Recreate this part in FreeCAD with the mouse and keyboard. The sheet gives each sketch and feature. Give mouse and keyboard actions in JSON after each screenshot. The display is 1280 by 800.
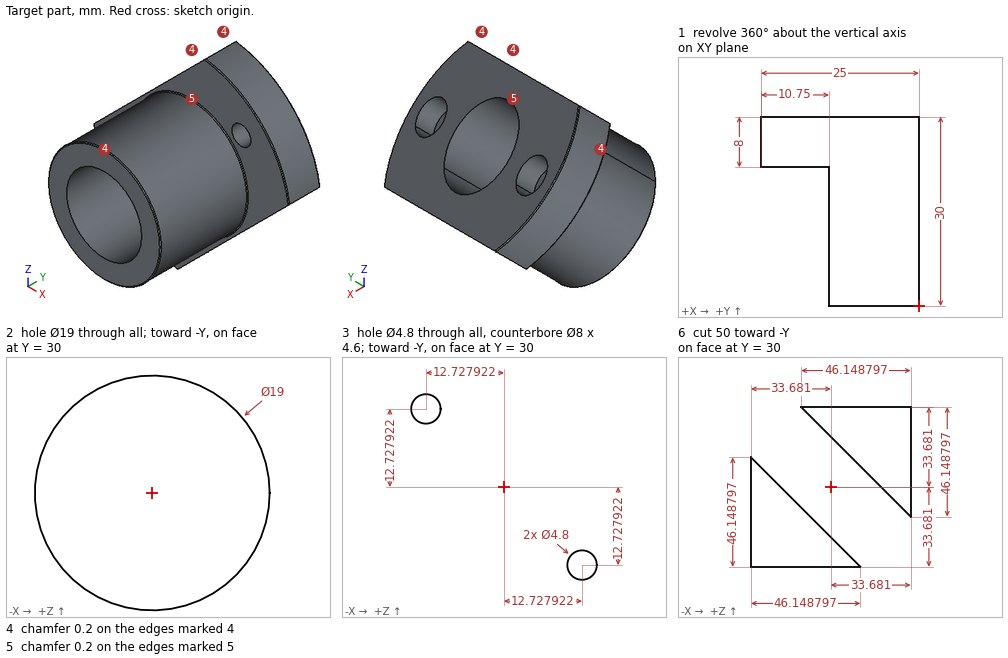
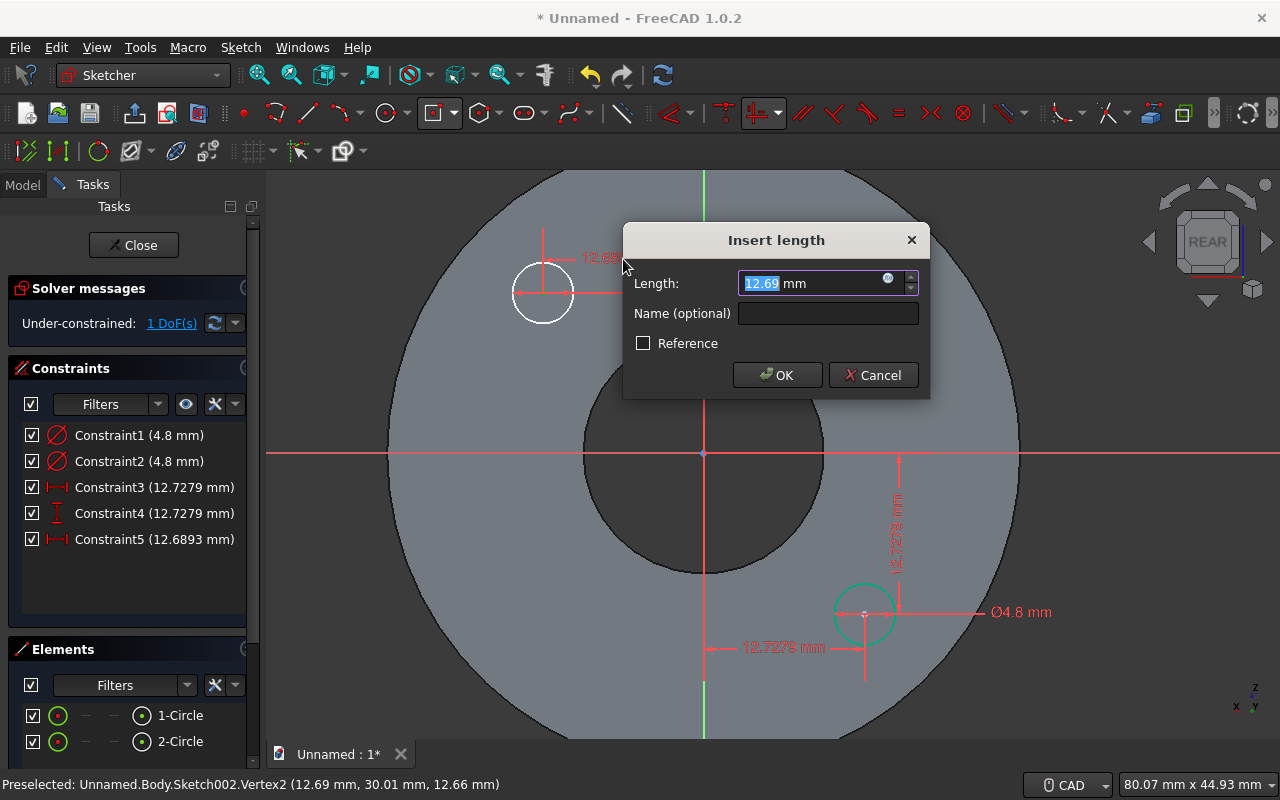
{"action": "type", "text": "12.727922"}
{"action": "key", "text": "Return"}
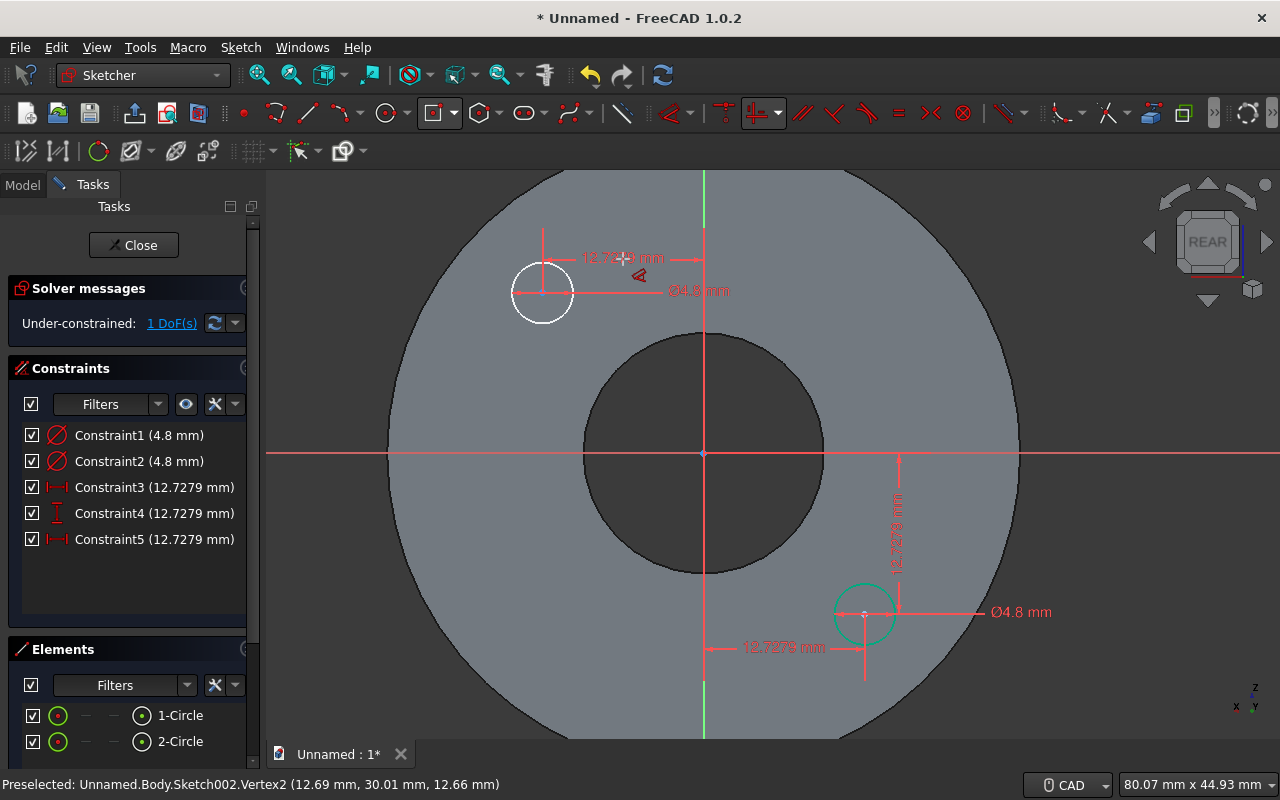
{"action": "left_click", "coordinate": [543, 293]}
{"action": "left_click", "coordinate": [509, 373]}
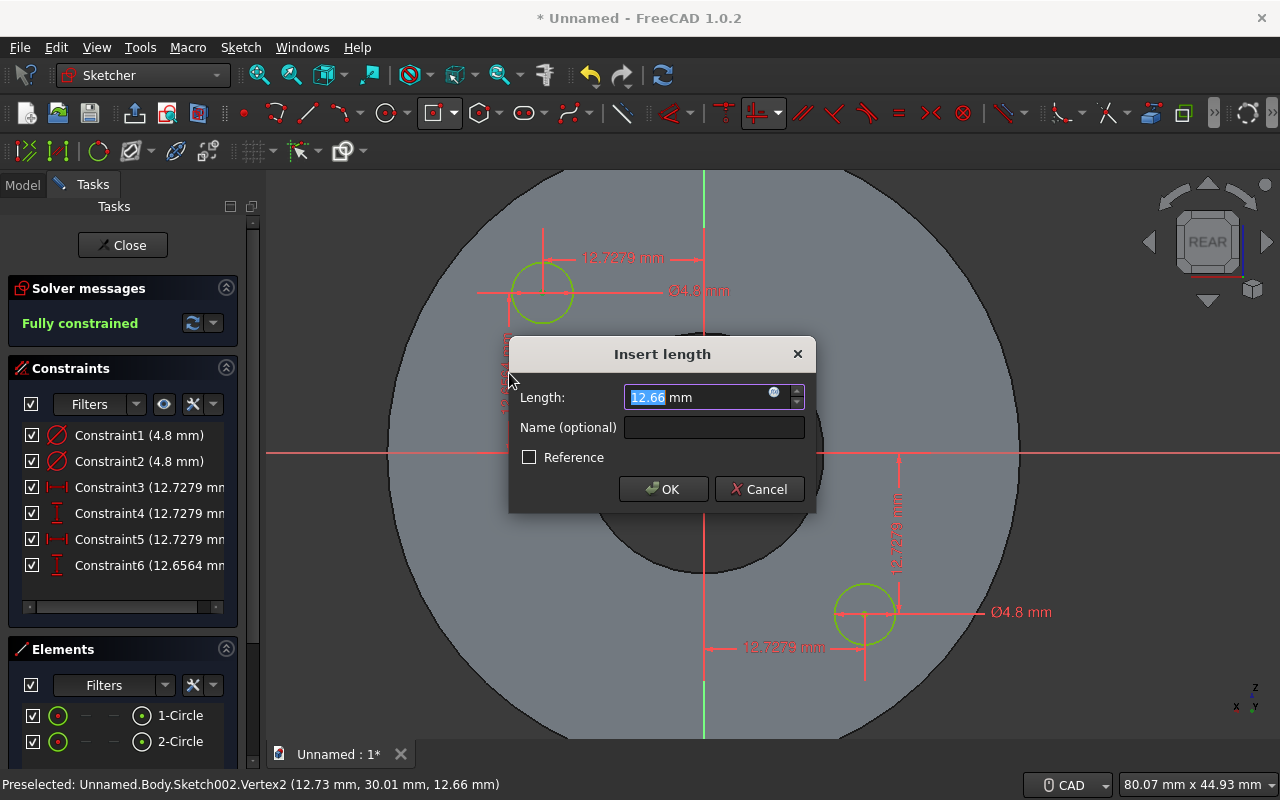
{"action": "type", "text": "12.727922"}
{"action": "key", "text": "Return"}
{"action": "key", "text": "Escape"}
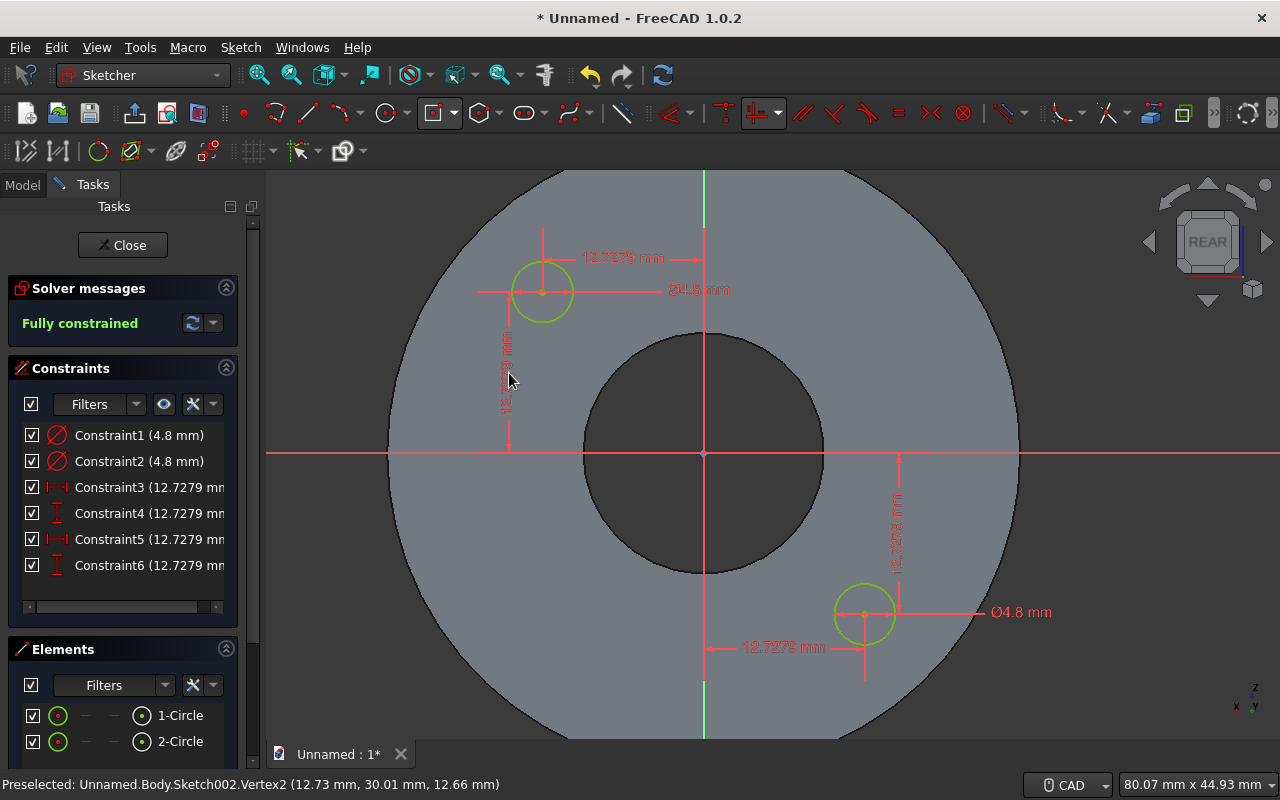
{"action": "left_click", "coordinate": [123, 245]}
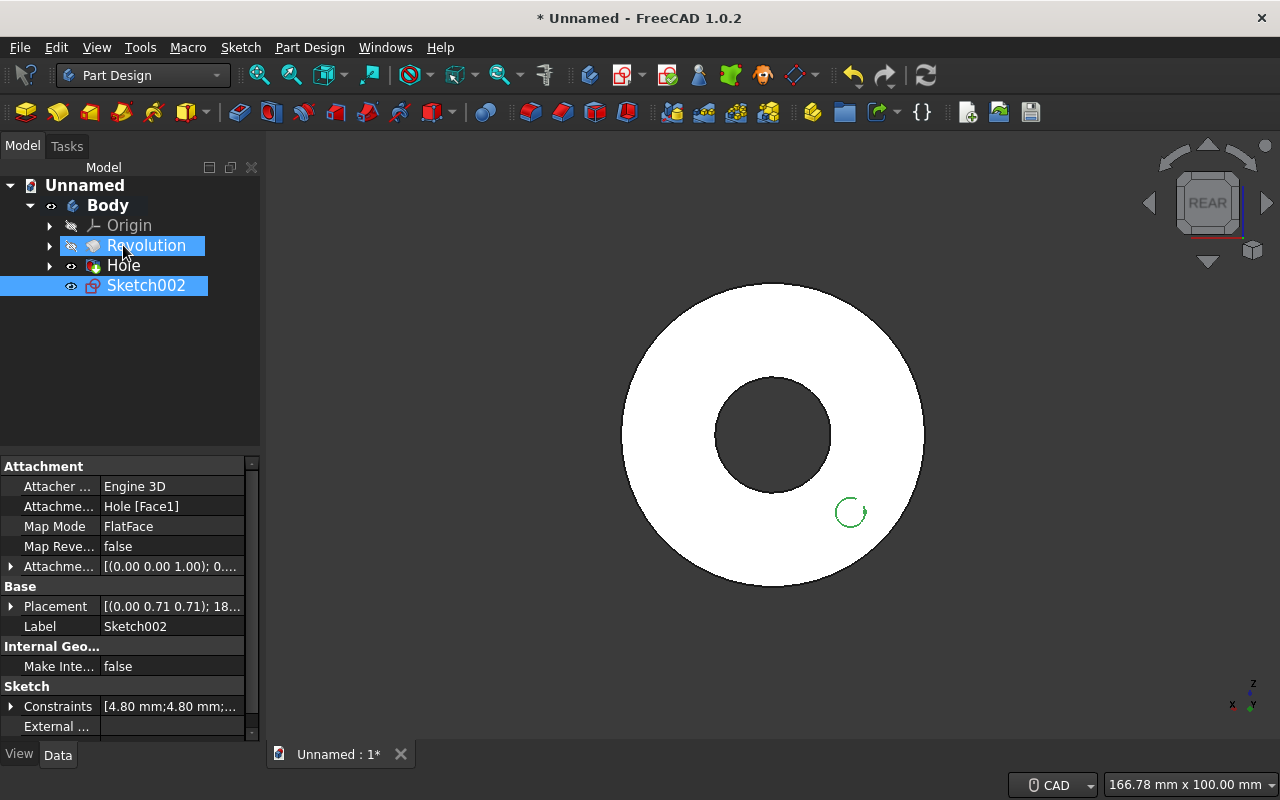
{"action": "left_click", "coordinate": [272, 112]}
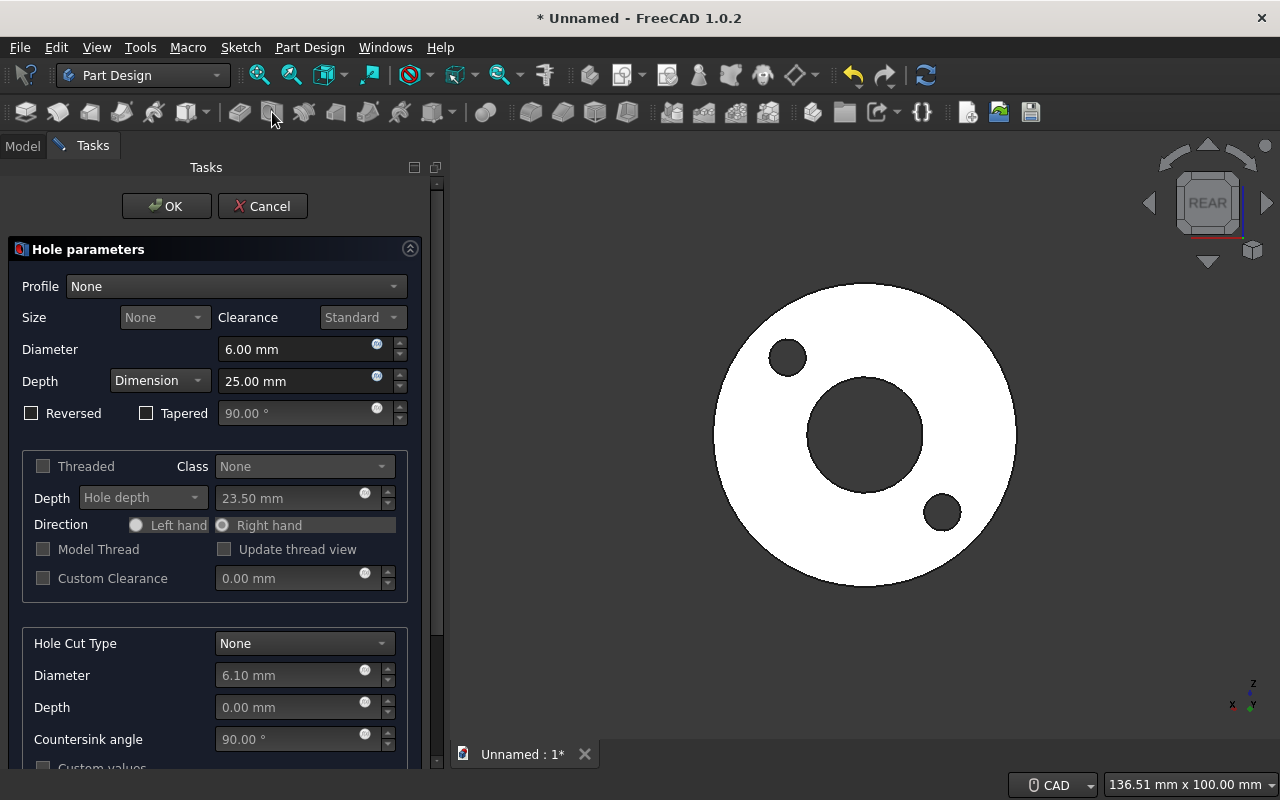
{"action": "triple_click", "coordinate": [305, 349]}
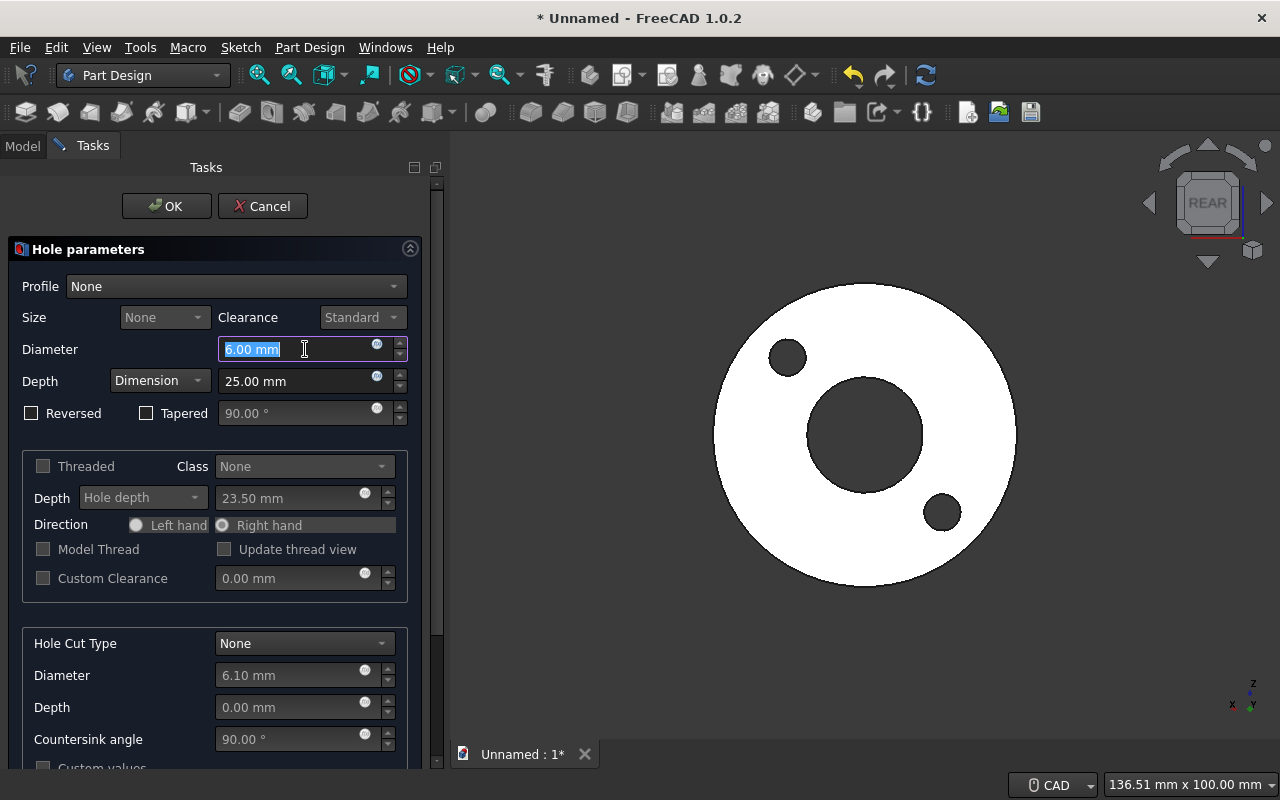
{"action": "type", "text": "4.8"}
{"action": "key", "text": "Tab"}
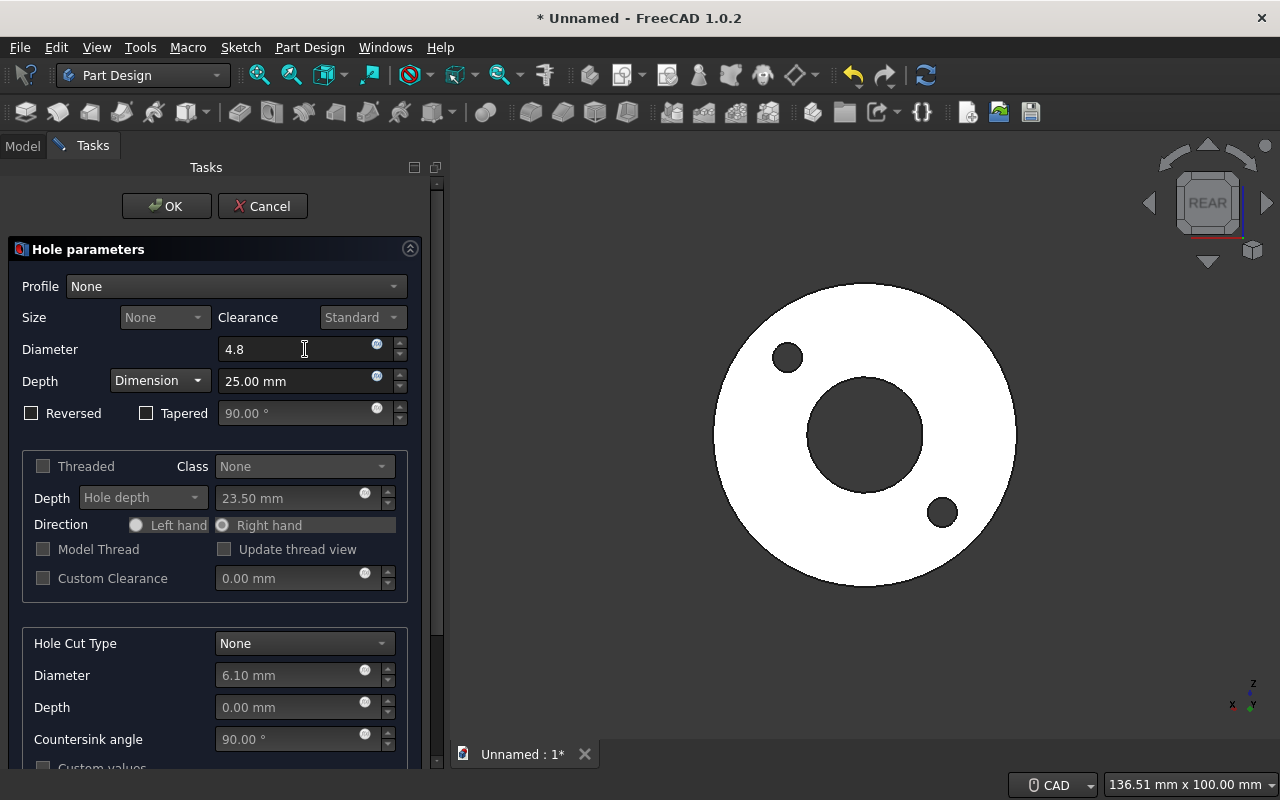
{"action": "left_click", "coordinate": [161, 380]}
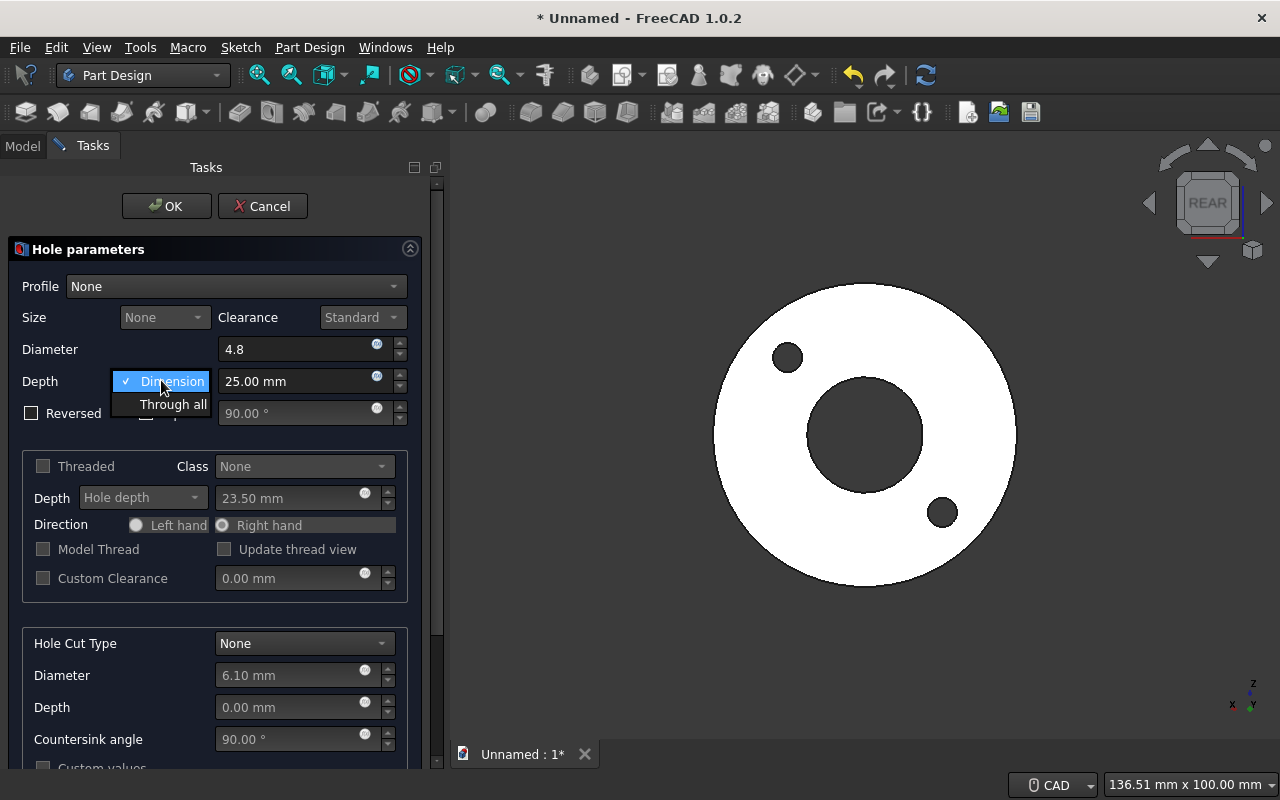
{"action": "left_click", "coordinate": [160, 404]}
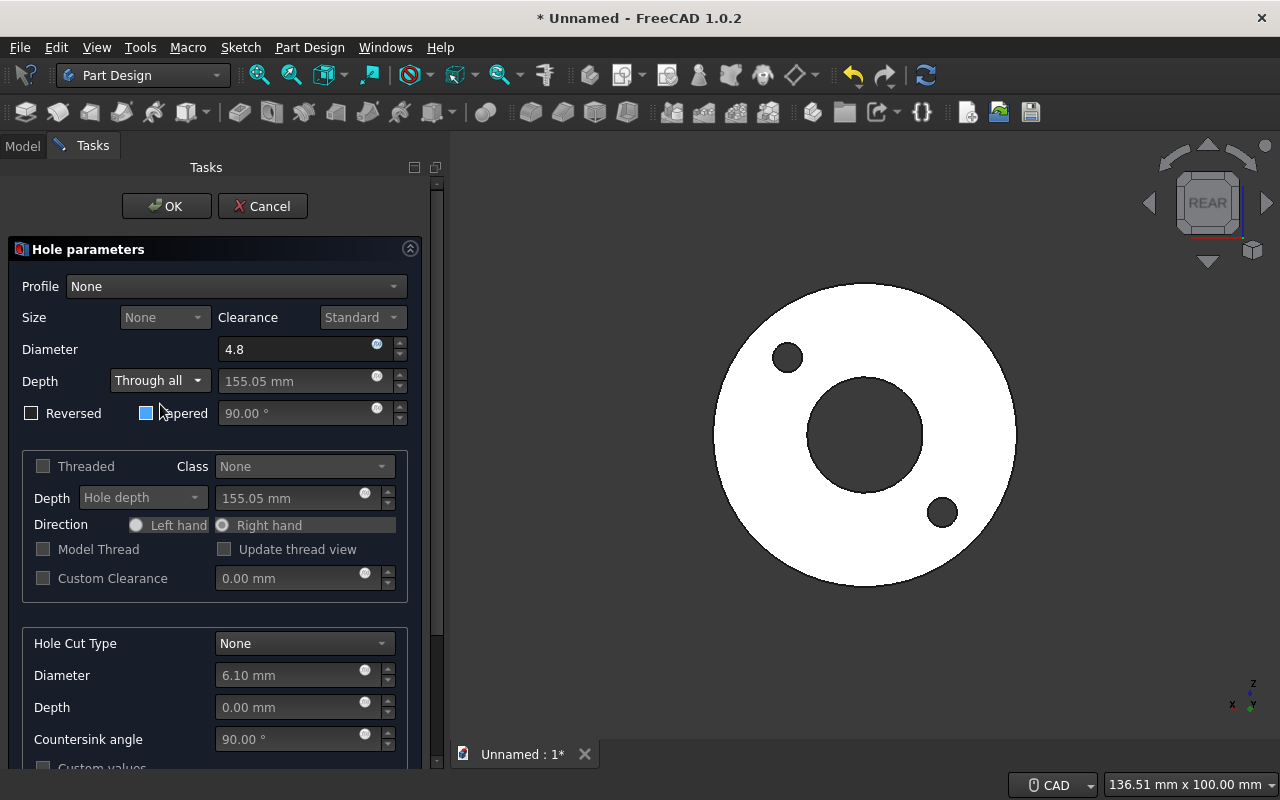
{"action": "left_click", "coordinate": [306, 644]}